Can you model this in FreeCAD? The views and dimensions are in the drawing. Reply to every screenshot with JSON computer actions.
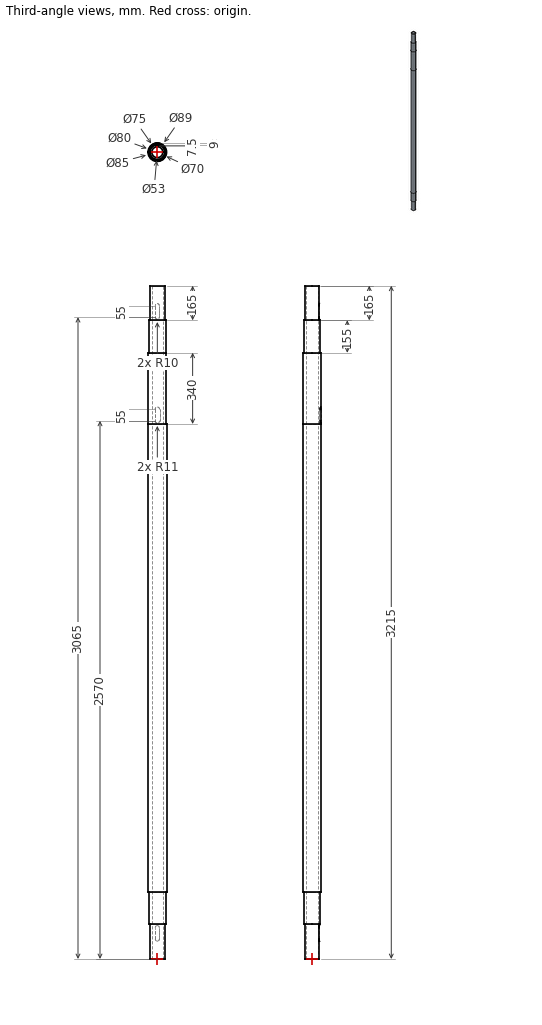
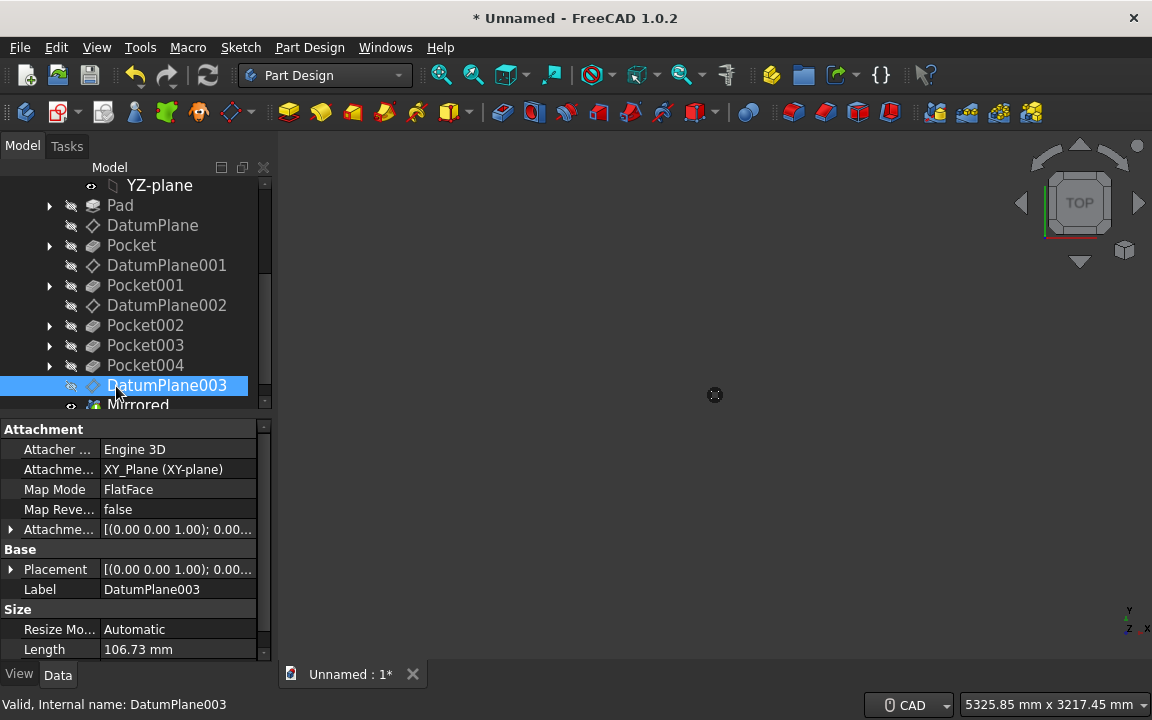
{"action": "left_click", "coordinate": [442, 76]}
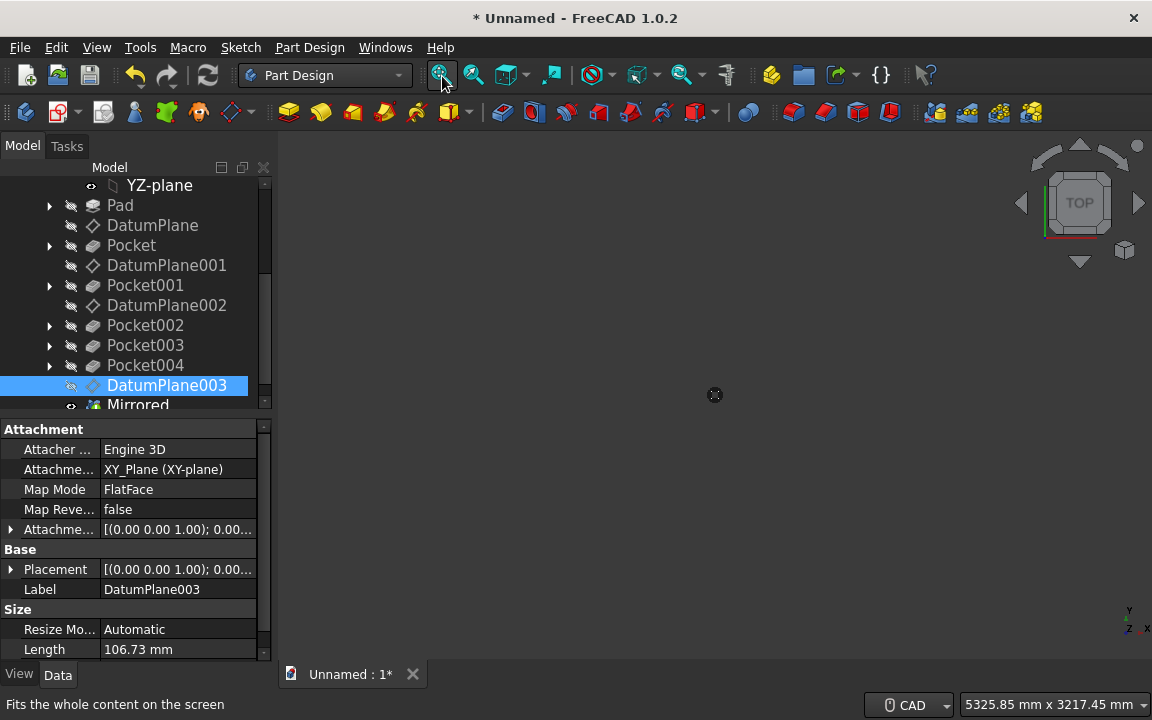
{"action": "scroll", "coordinate": [160, 301], "scroll_direction": "down", "scroll_amount": 3}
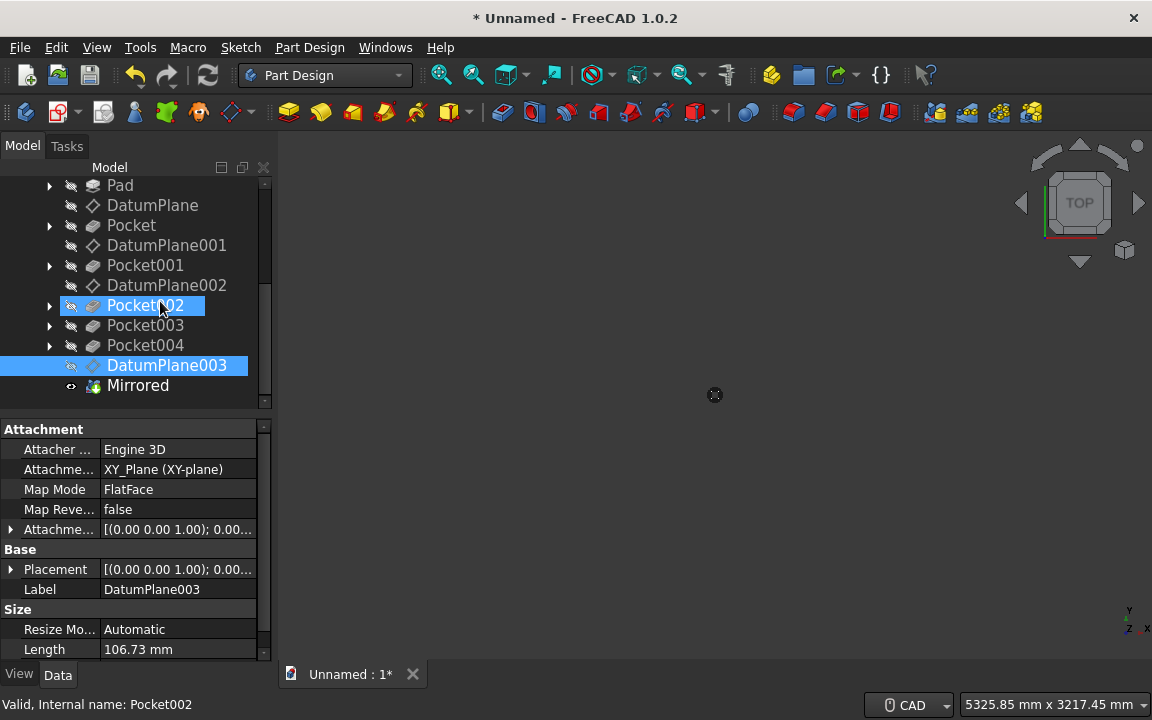
{"action": "scroll", "coordinate": [140, 281], "scroll_direction": "up", "scroll_amount": 15}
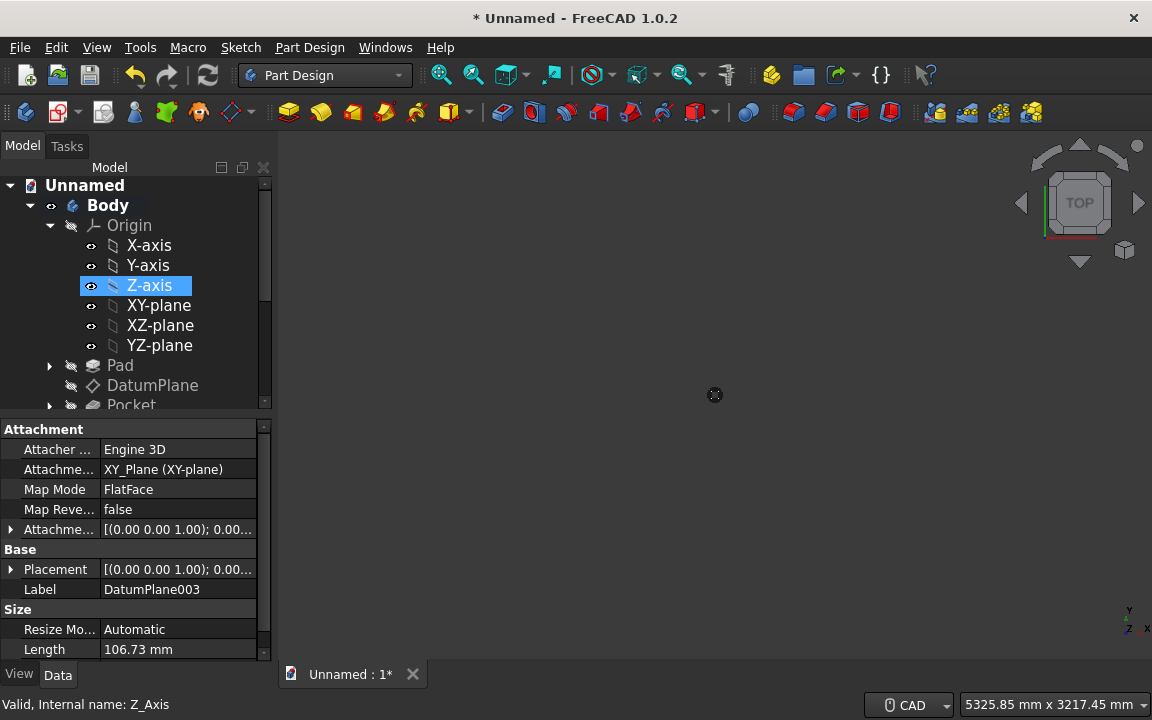
{"action": "left_click", "coordinate": [136, 326]}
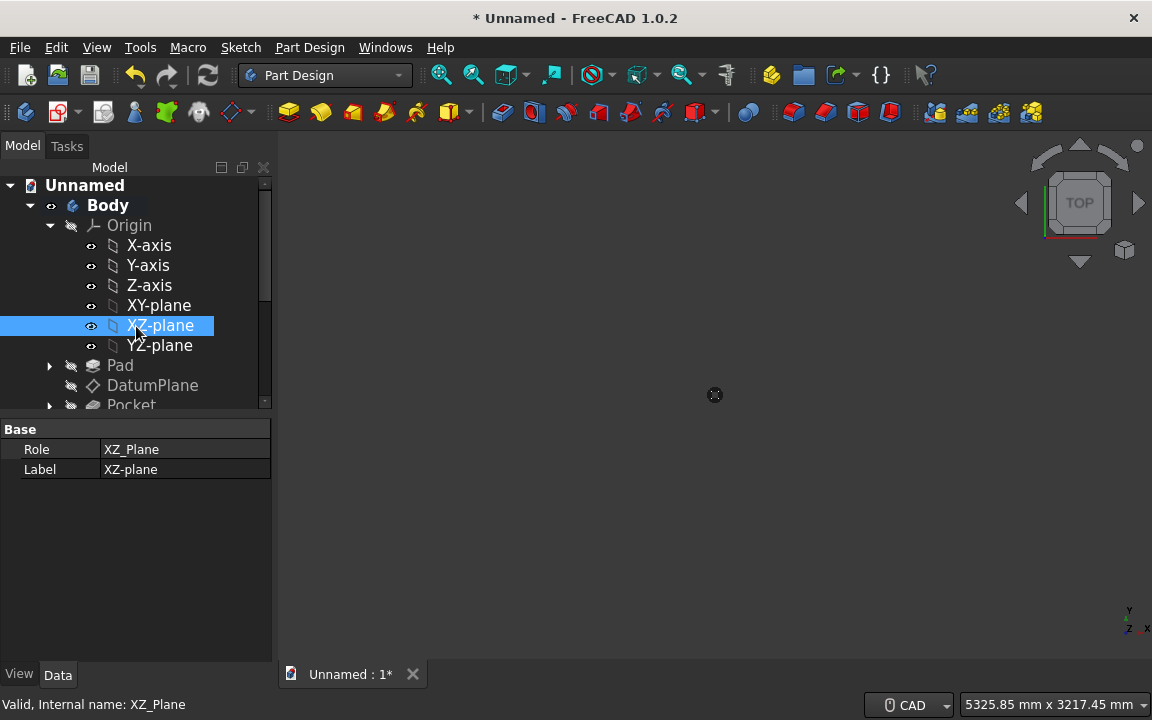
{"action": "left_click", "coordinate": [232, 112]}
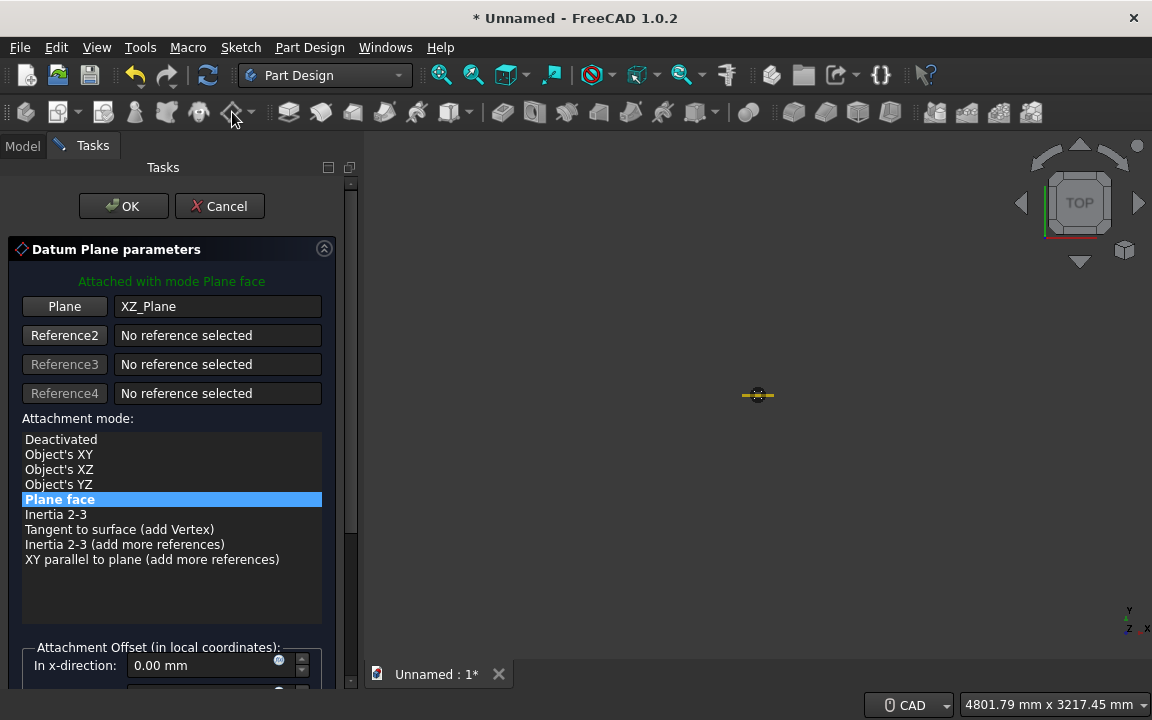
{"action": "scroll", "coordinate": [351, 432], "scroll_direction": "down", "scroll_amount": 2}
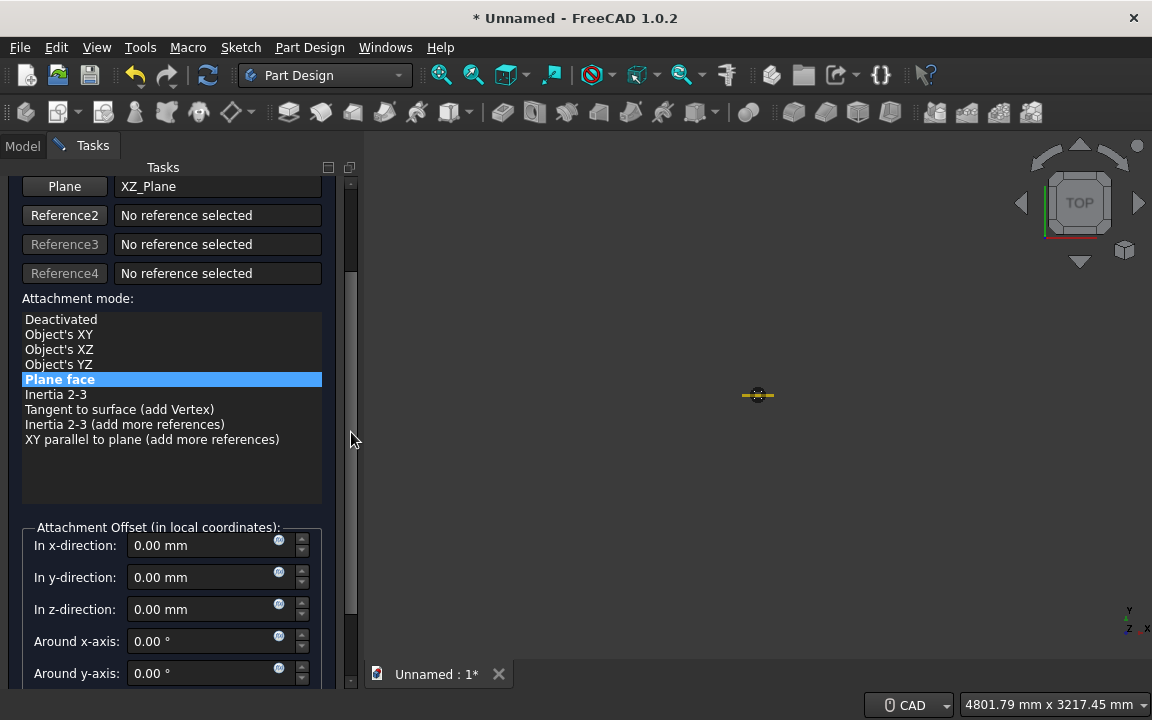
{"action": "triple_click", "coordinate": [210, 609]}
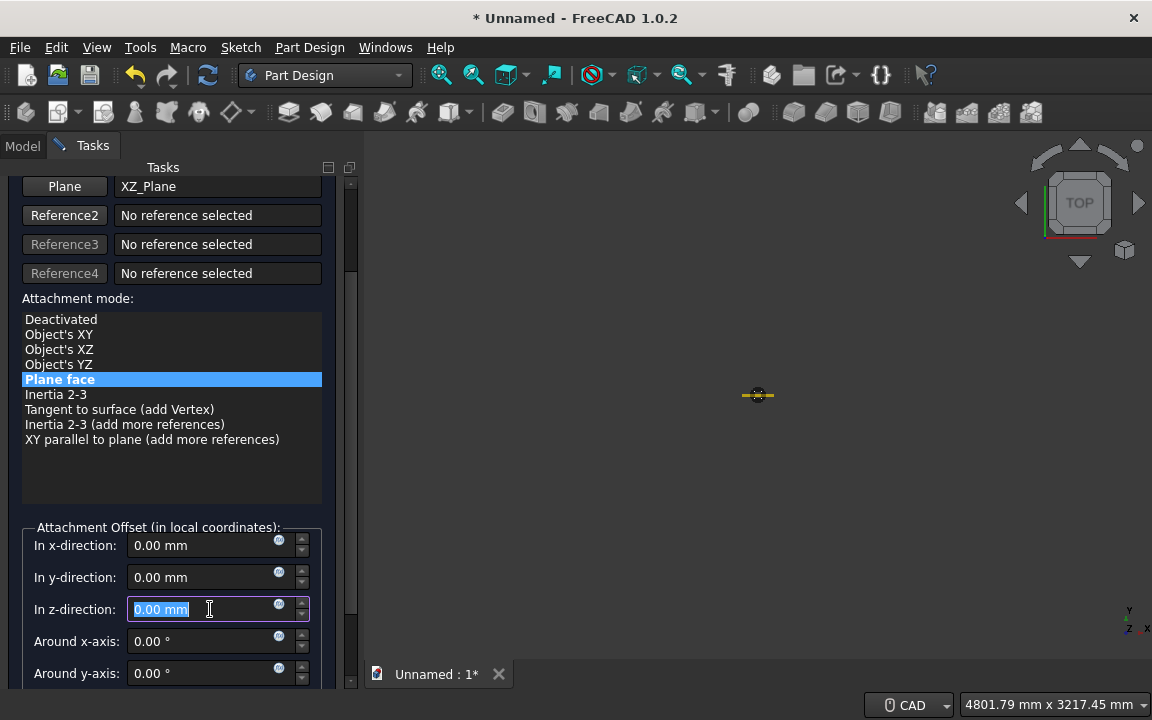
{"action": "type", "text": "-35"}
{"action": "key", "text": "Tab"}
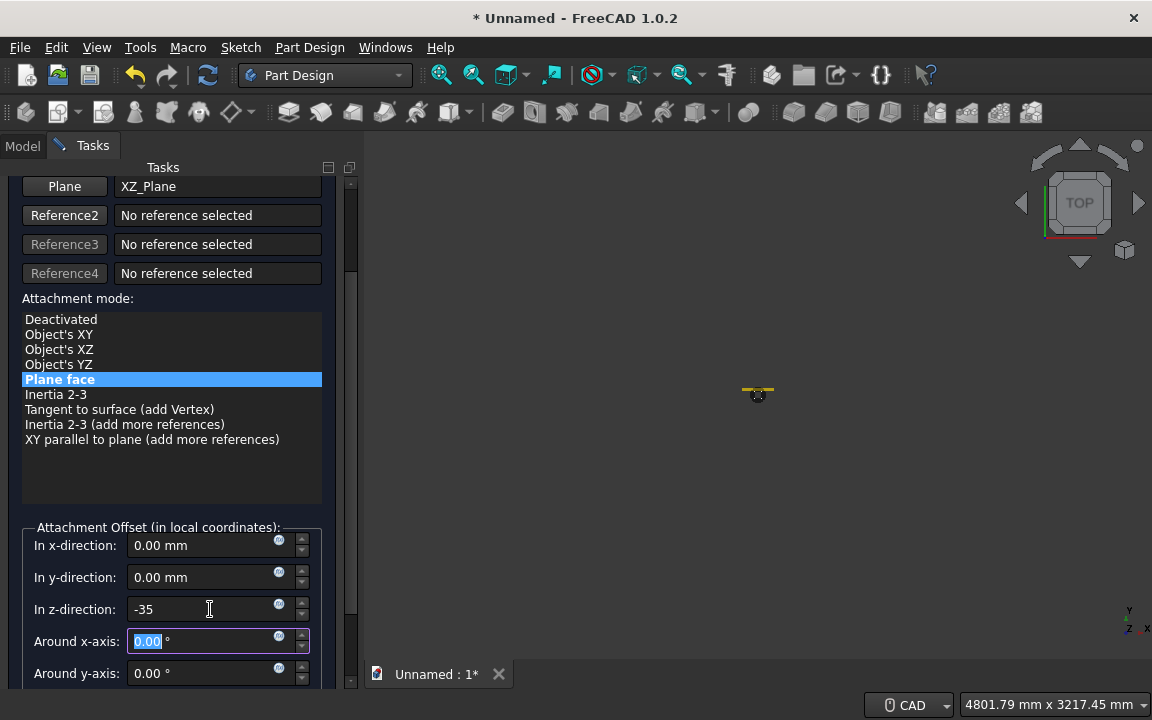
{"action": "scroll", "coordinate": [351, 432], "scroll_direction": "up", "scroll_amount": 3}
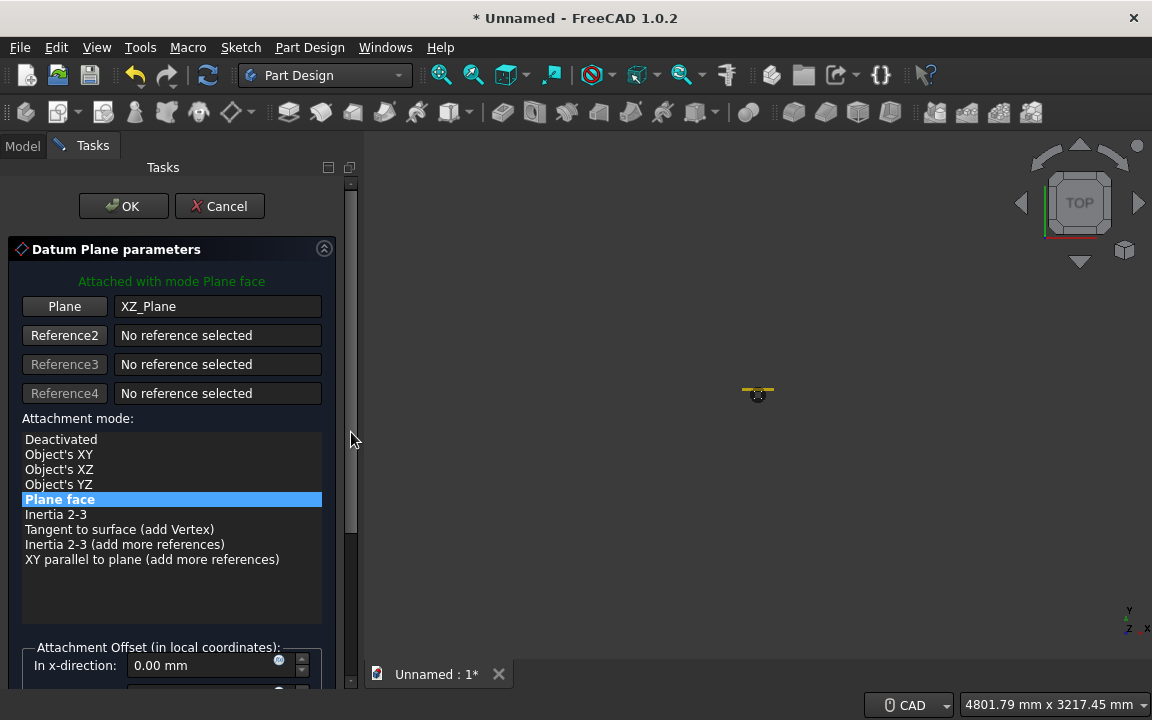
{"action": "left_click", "coordinate": [124, 206]}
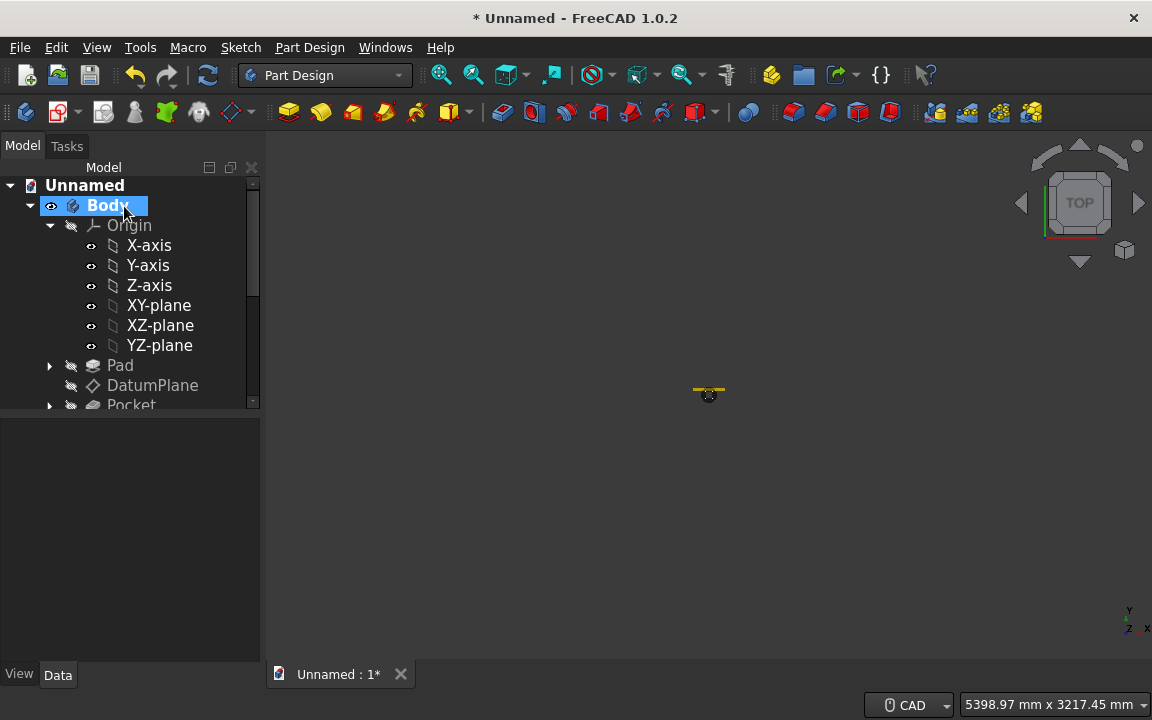
{"action": "scroll", "coordinate": [100, 301], "scroll_direction": "down", "scroll_amount": 3}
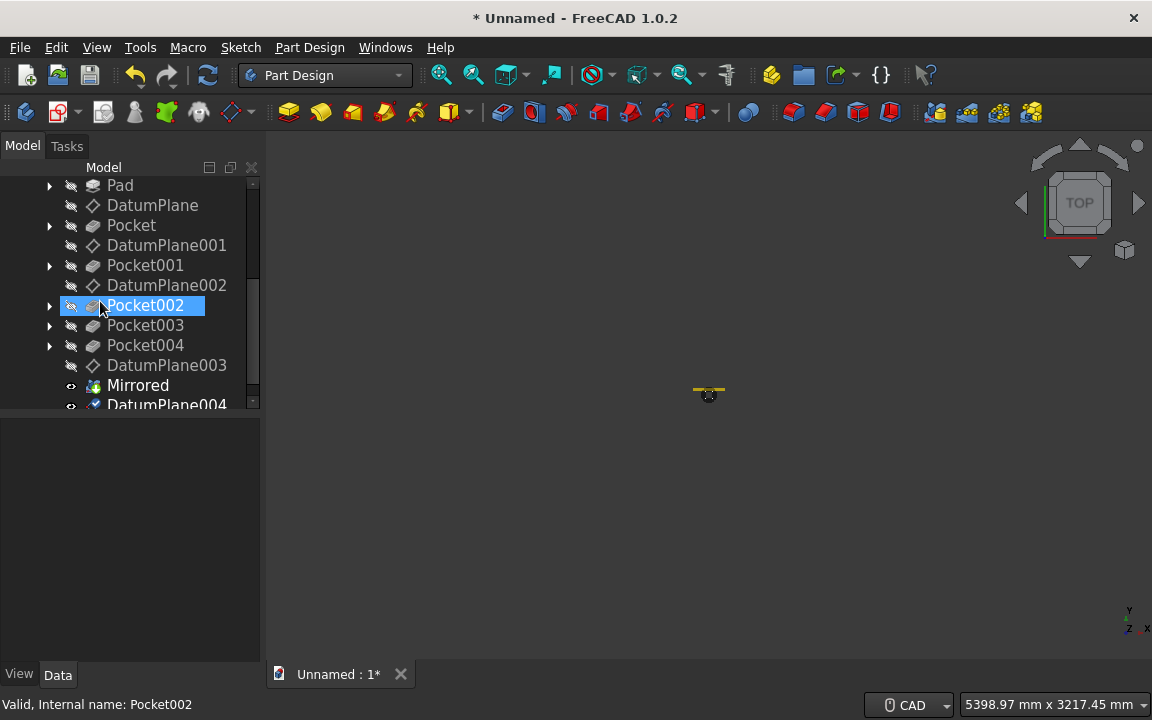
{"action": "left_click", "coordinate": [116, 406]}